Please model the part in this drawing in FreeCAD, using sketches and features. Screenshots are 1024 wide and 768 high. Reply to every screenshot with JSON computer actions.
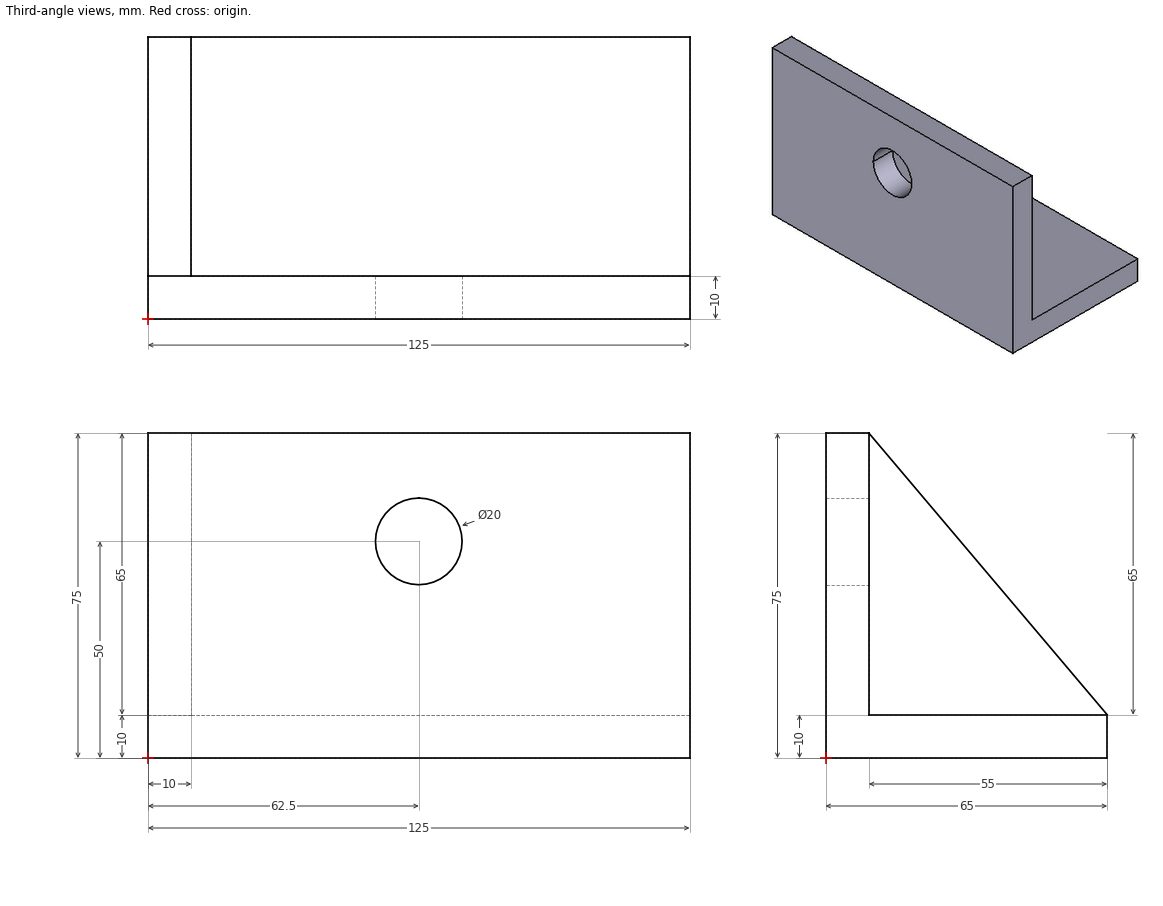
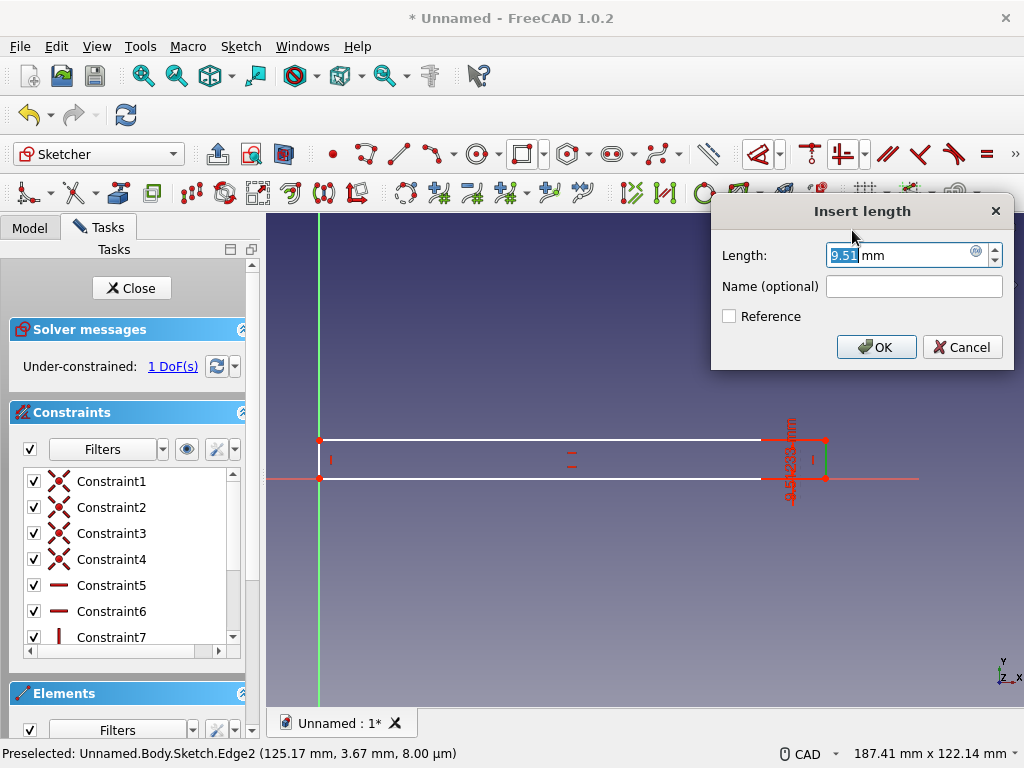
{"action": "type", "text": "10"}
{"action": "key", "text": "Return"}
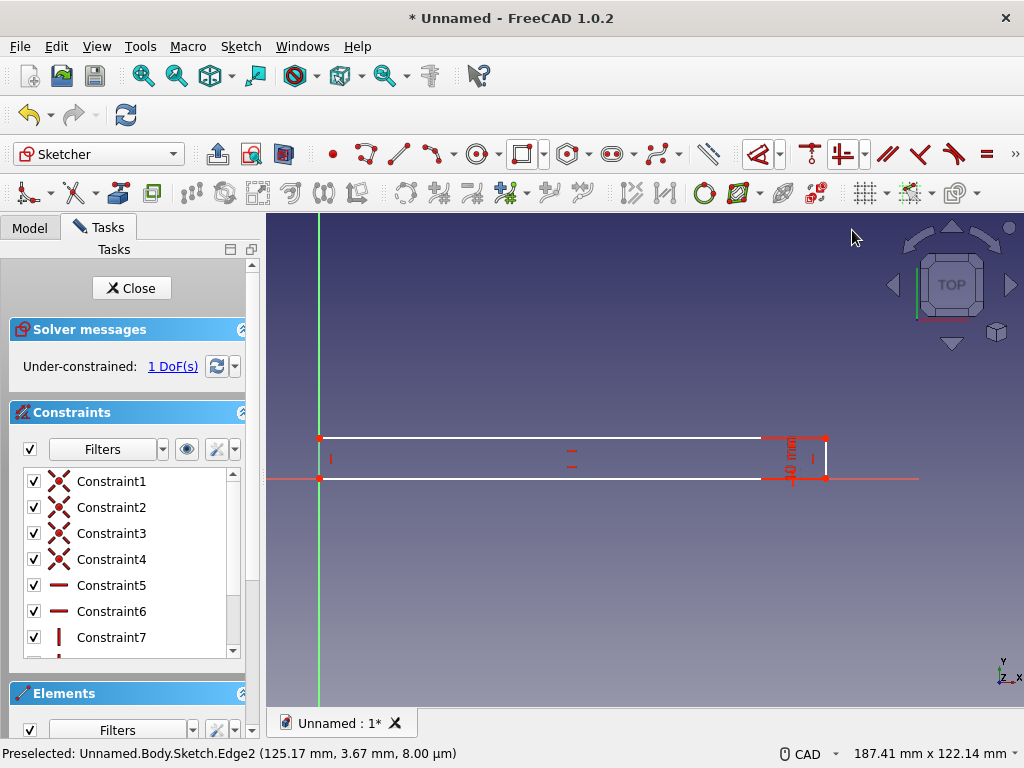
{"action": "left_click", "coordinate": [471, 479]}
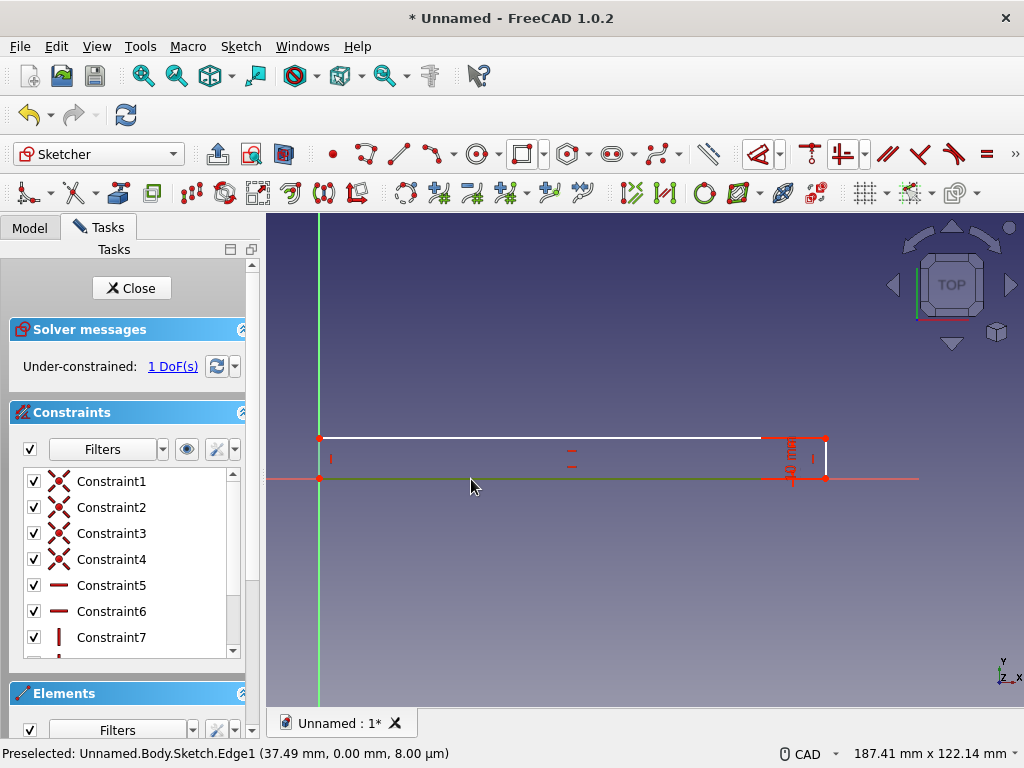
{"action": "left_click", "coordinate": [780, 154]}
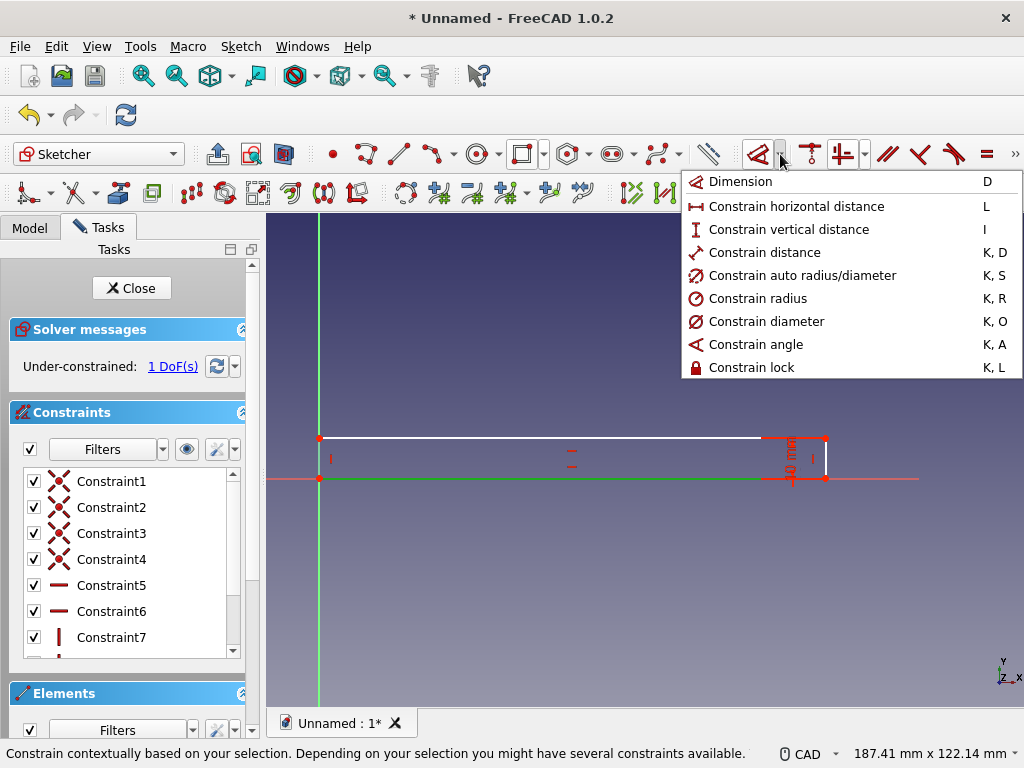
{"action": "left_click", "coordinate": [852, 206]}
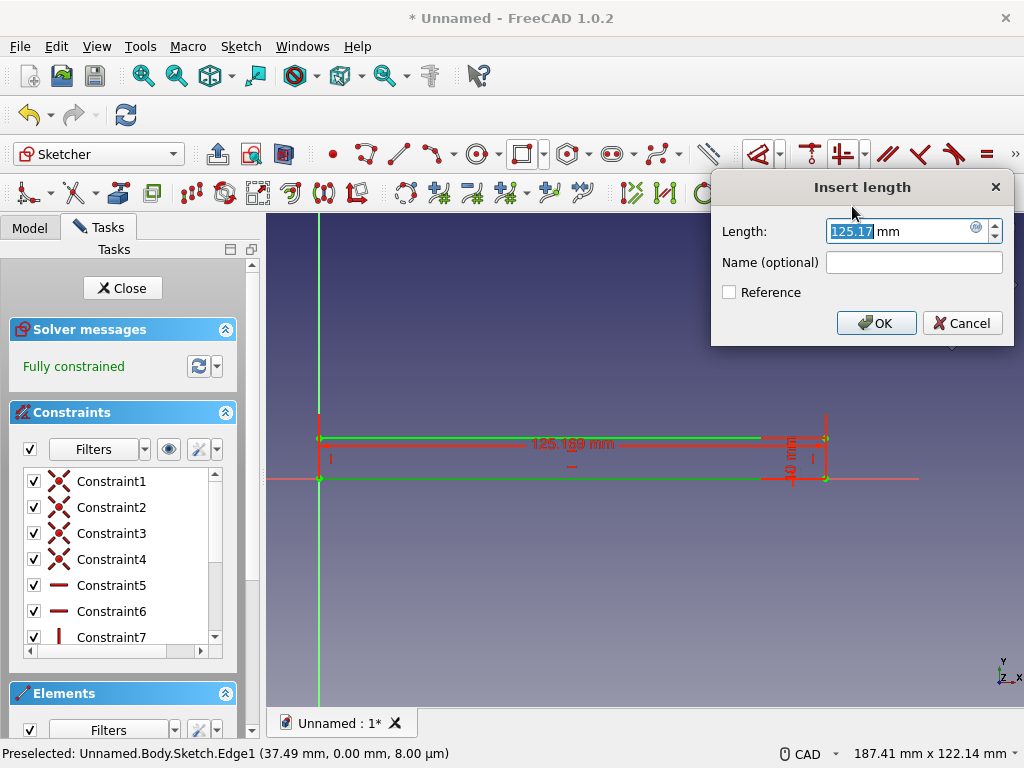
{"action": "type", "text": "125"}
{"action": "key", "text": "Return"}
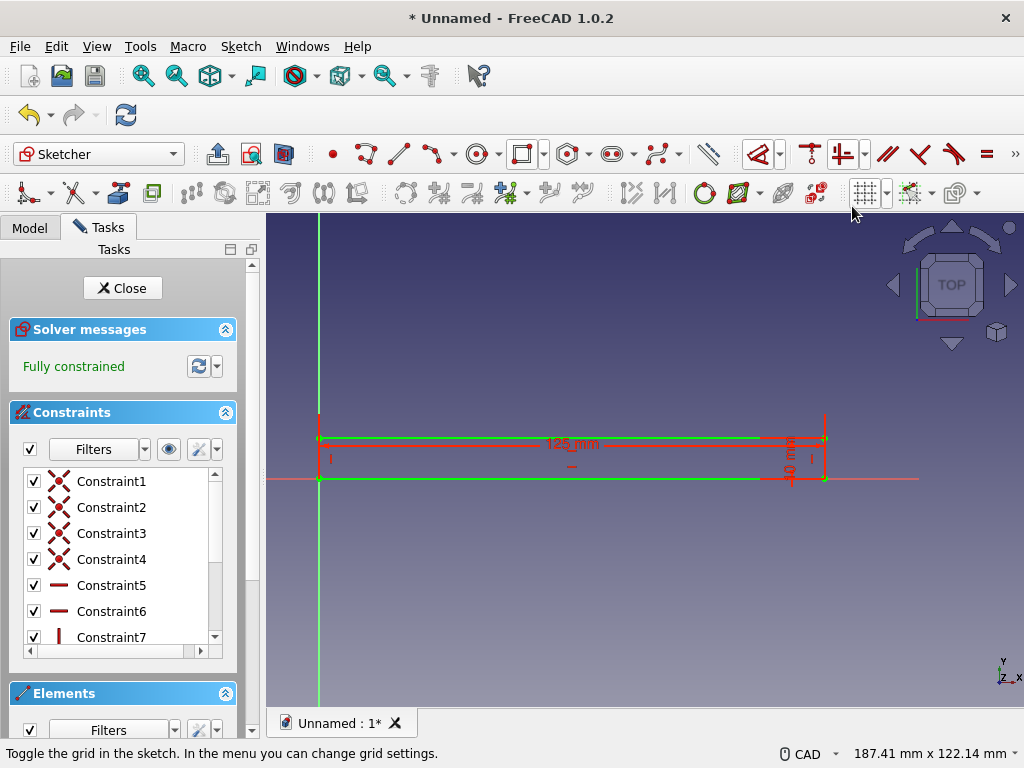
{"action": "left_click", "coordinate": [123, 288]}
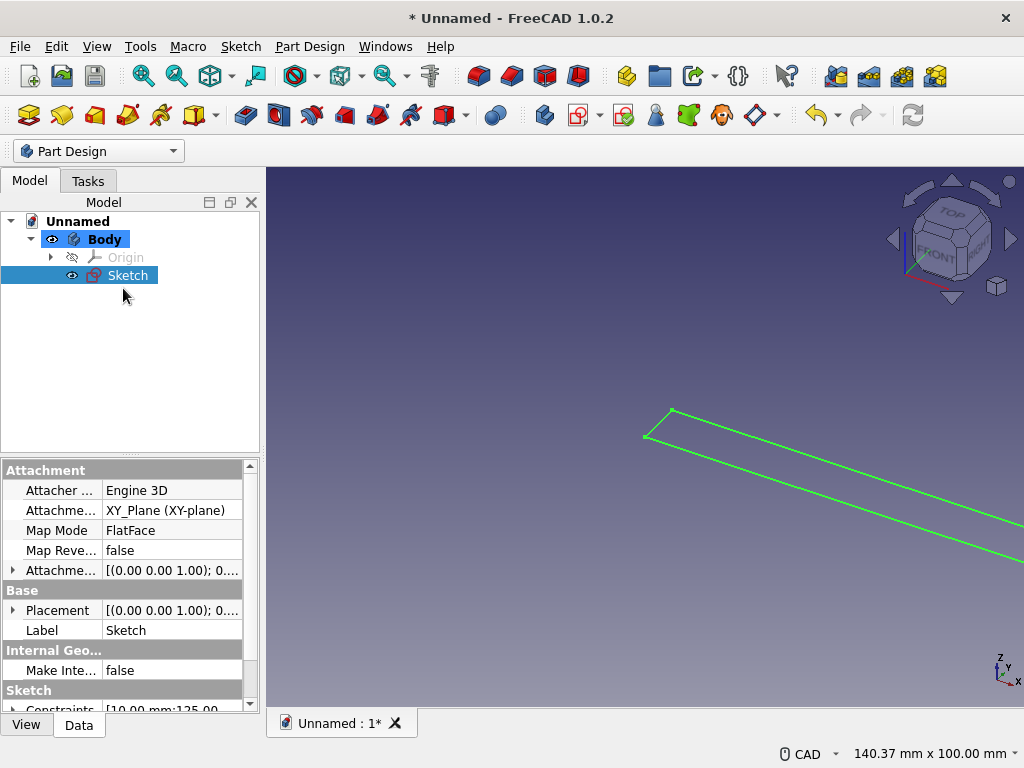
{"action": "left_click", "coordinate": [29, 116]}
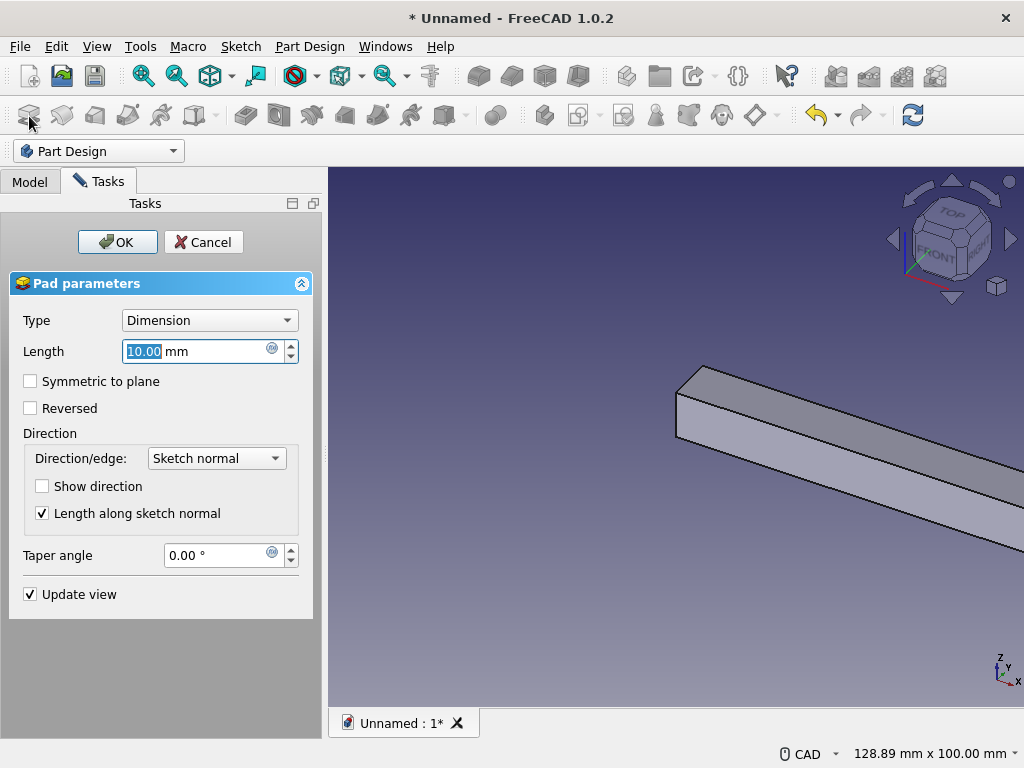
{"action": "type", "text": "75"}
{"action": "key", "text": "Tab"}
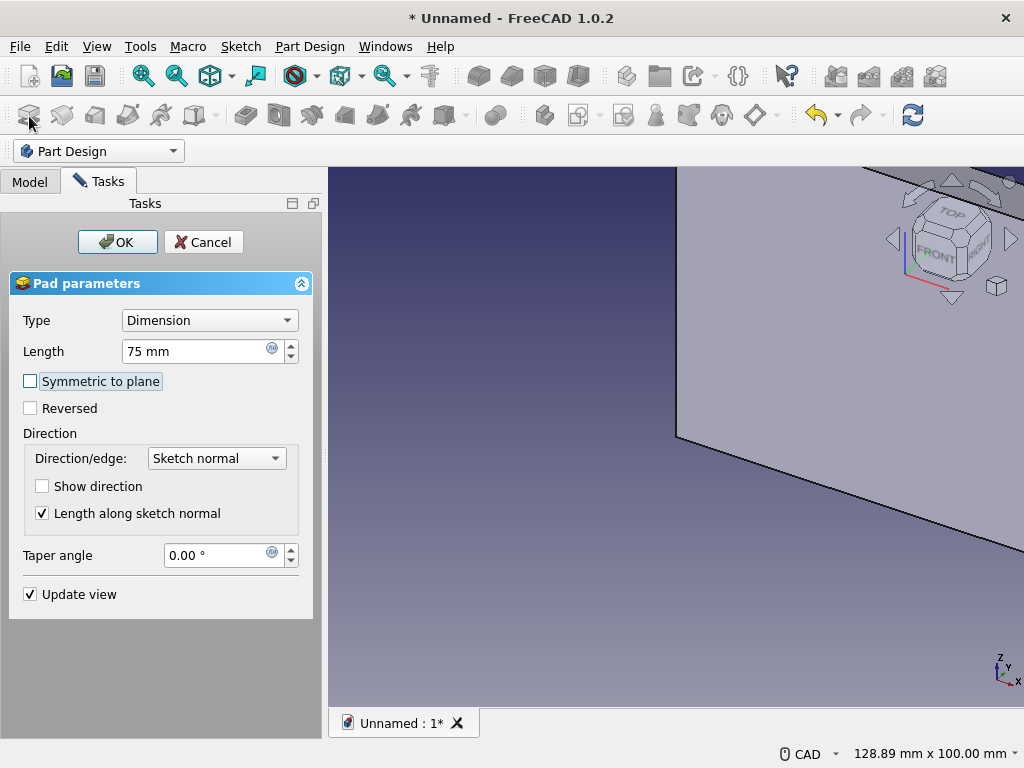
{"action": "left_click", "coordinate": [118, 242]}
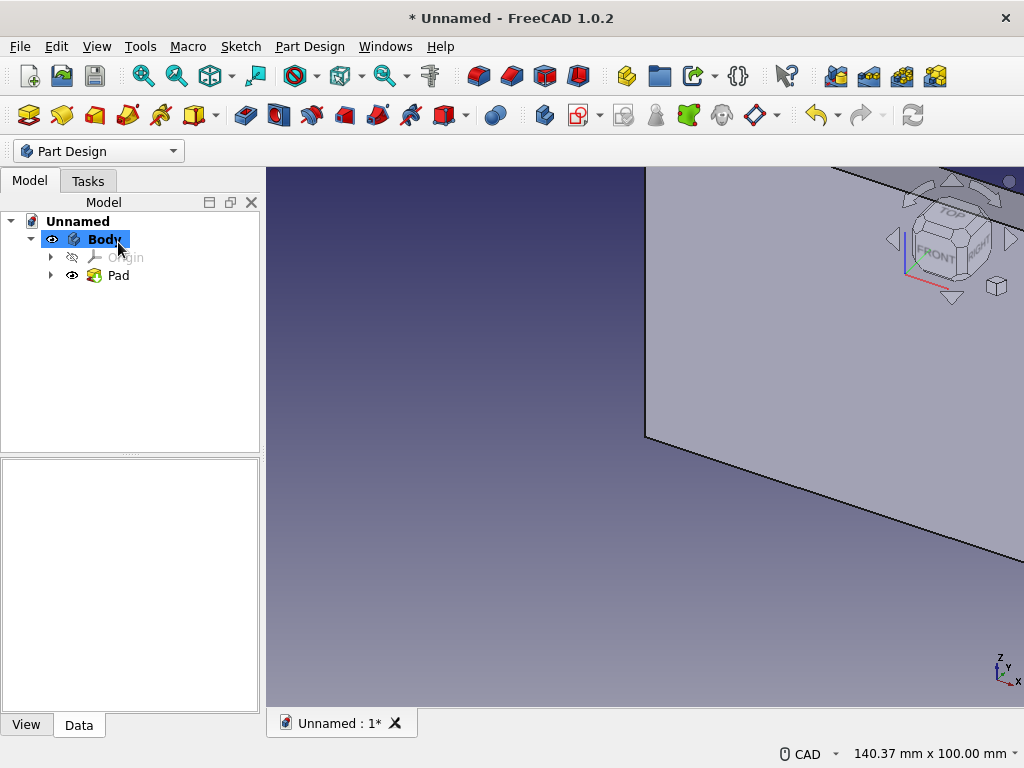
{"action": "left_click", "coordinate": [144, 76]}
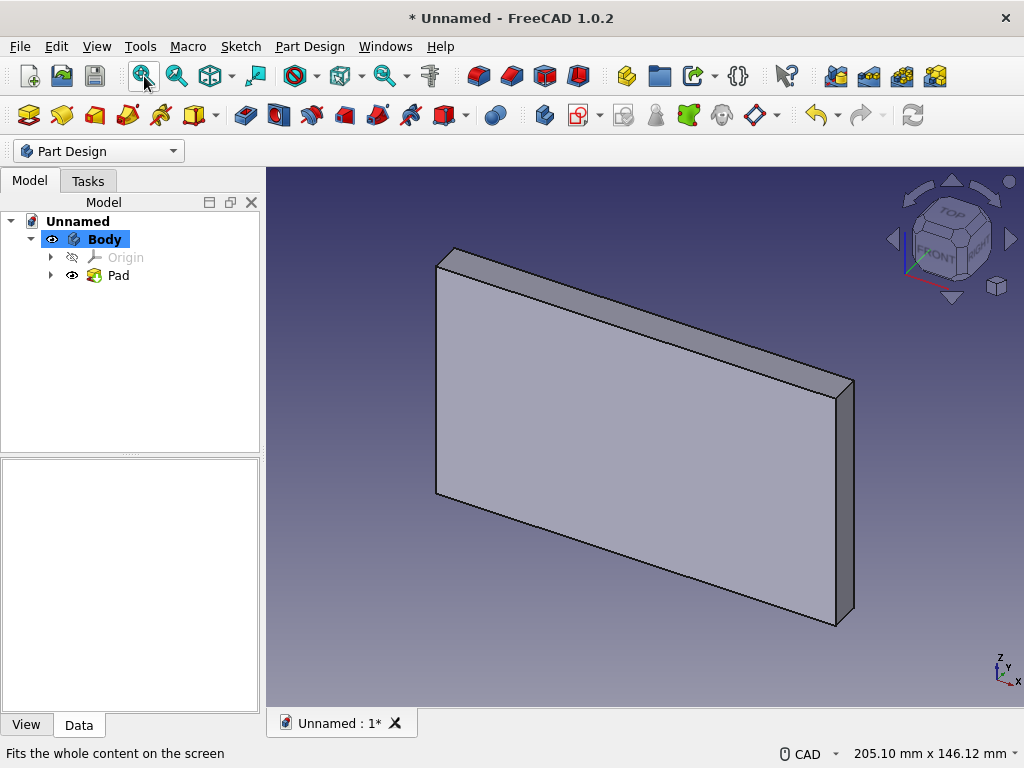
{"action": "key", "text": "4"}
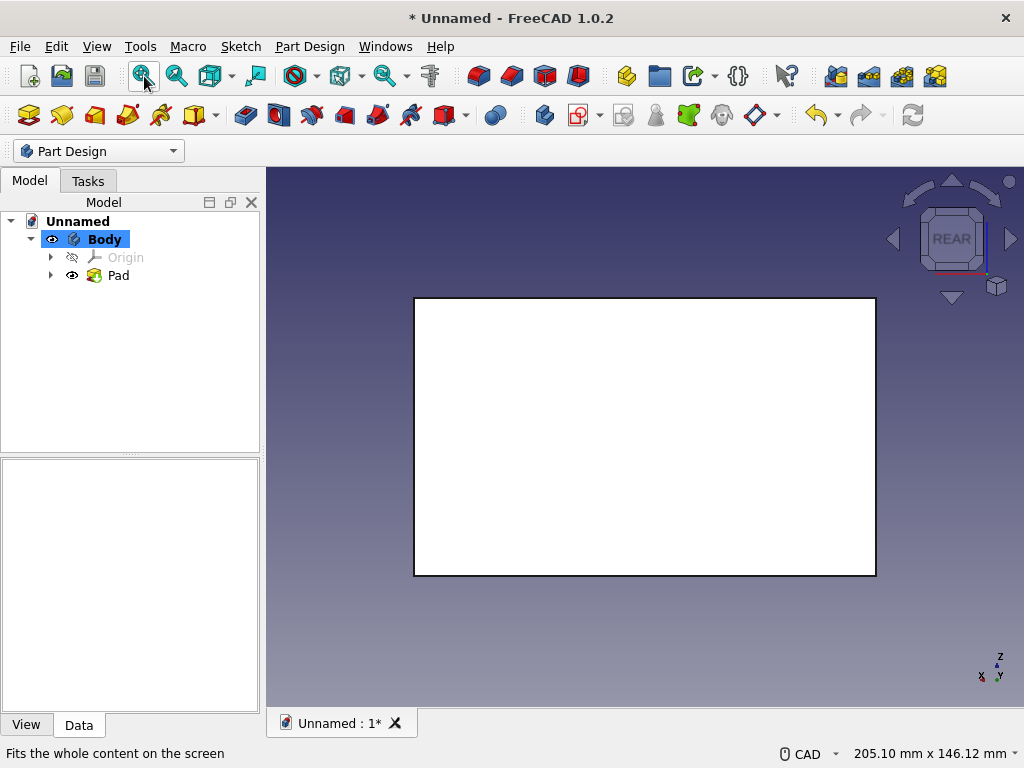
{"action": "left_click", "coordinate": [579, 436]}